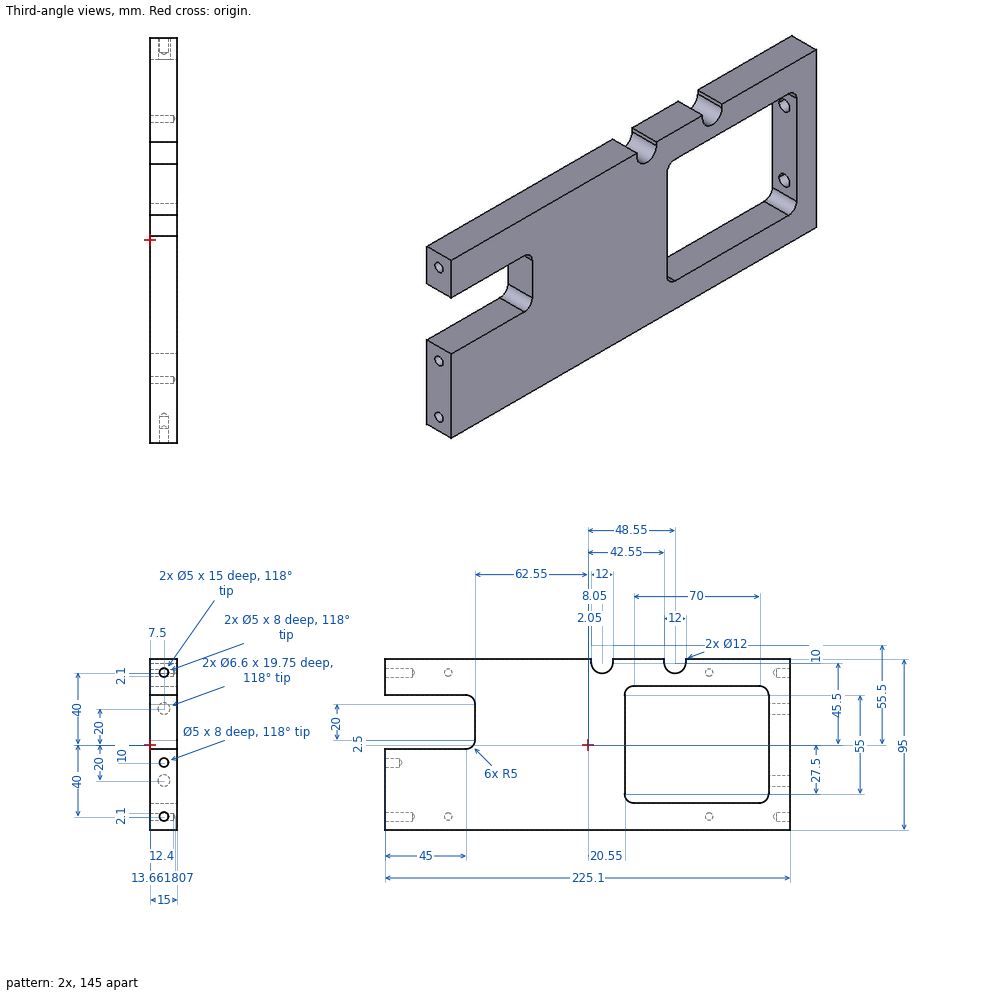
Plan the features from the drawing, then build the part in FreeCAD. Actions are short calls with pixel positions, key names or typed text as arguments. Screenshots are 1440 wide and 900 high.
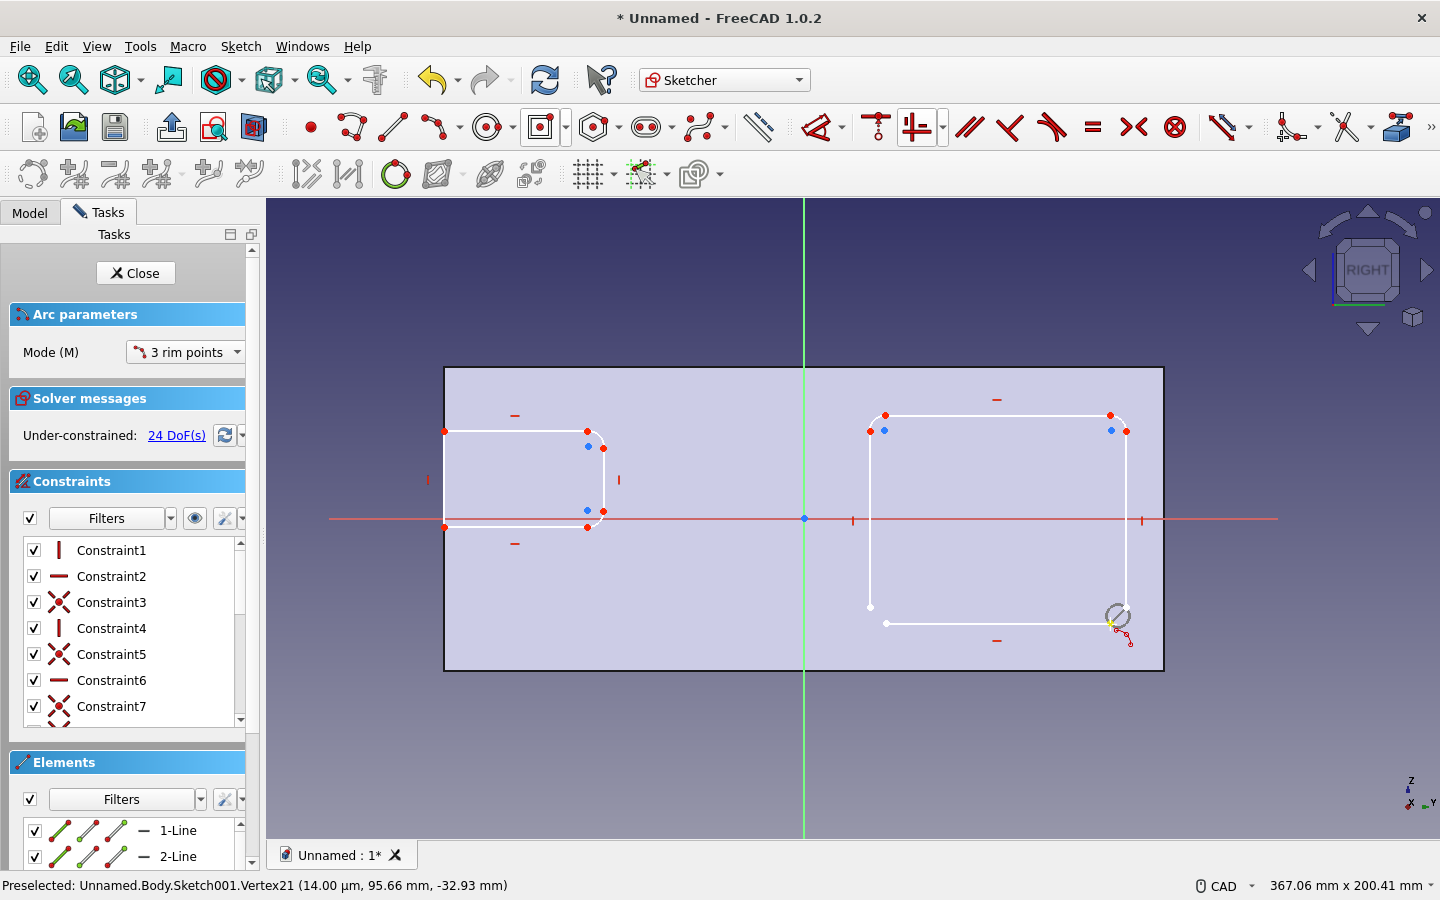
scroll(1121, 618, up, 7)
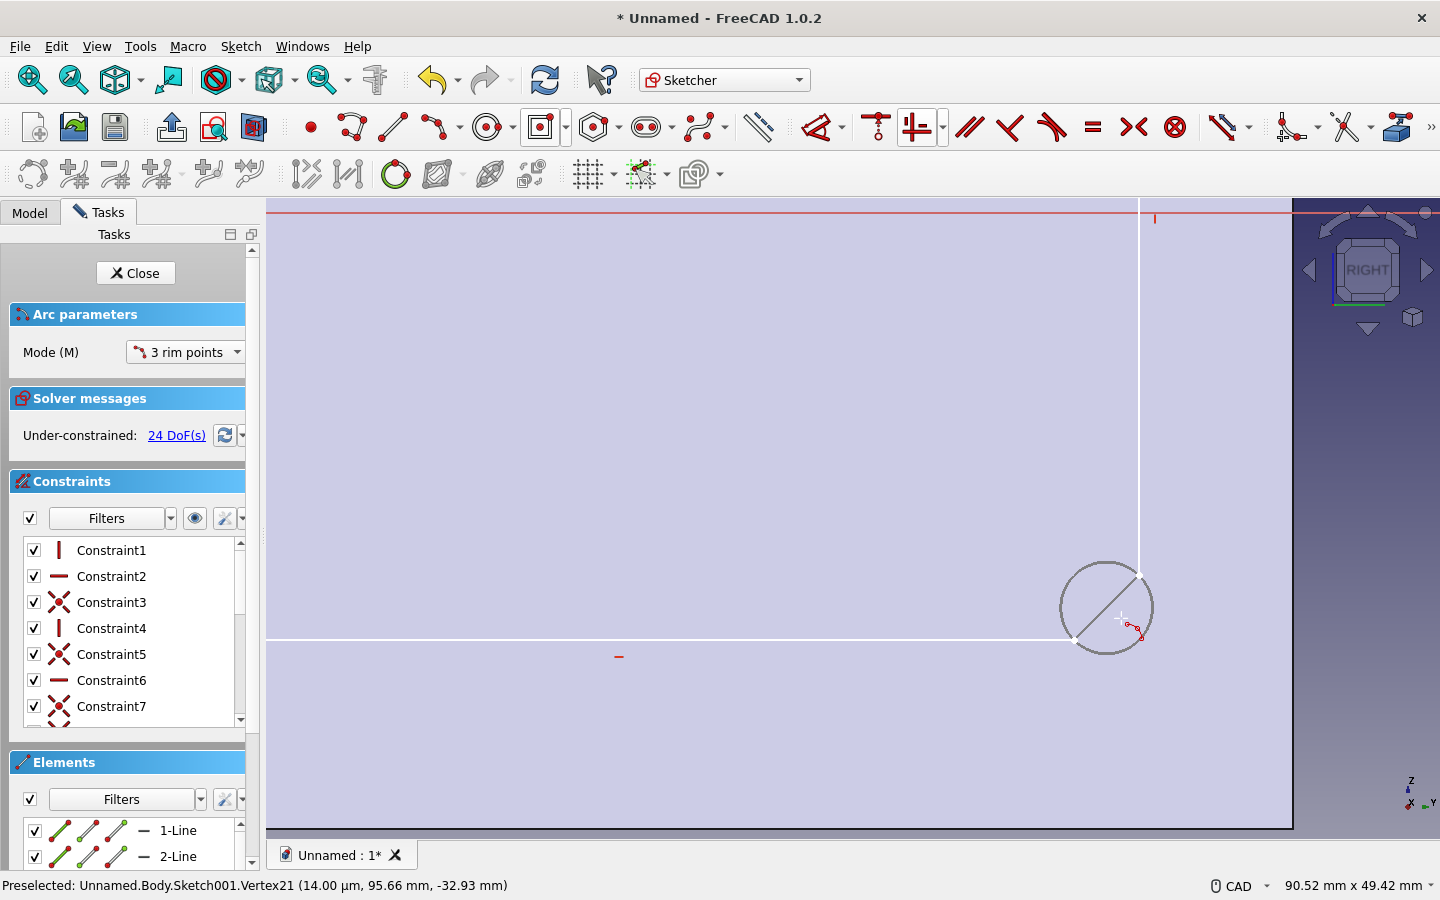
click(1119, 616)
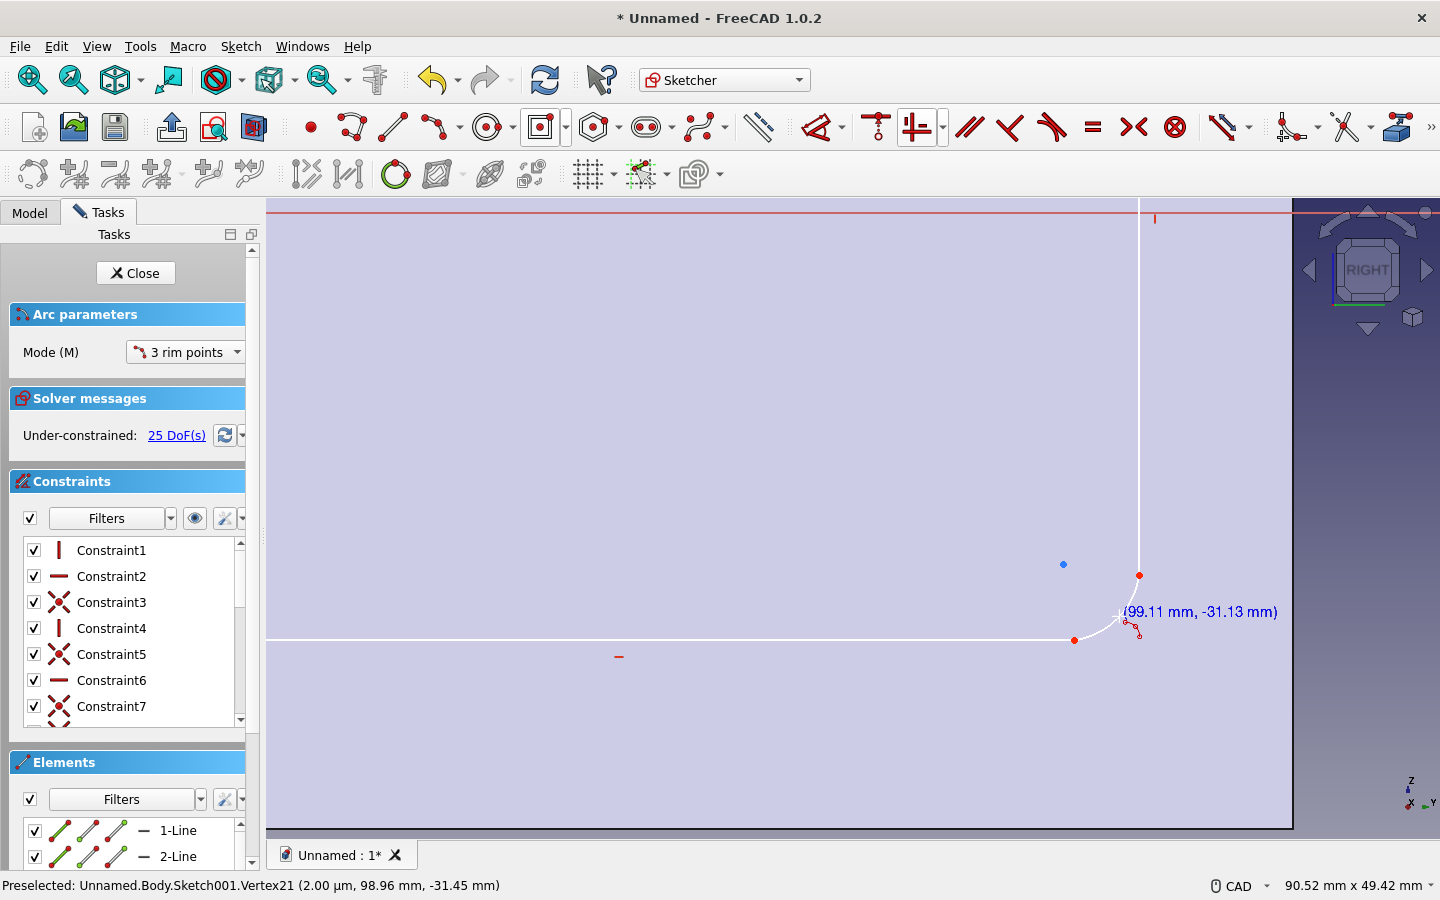
scroll(1121, 618, down, 7)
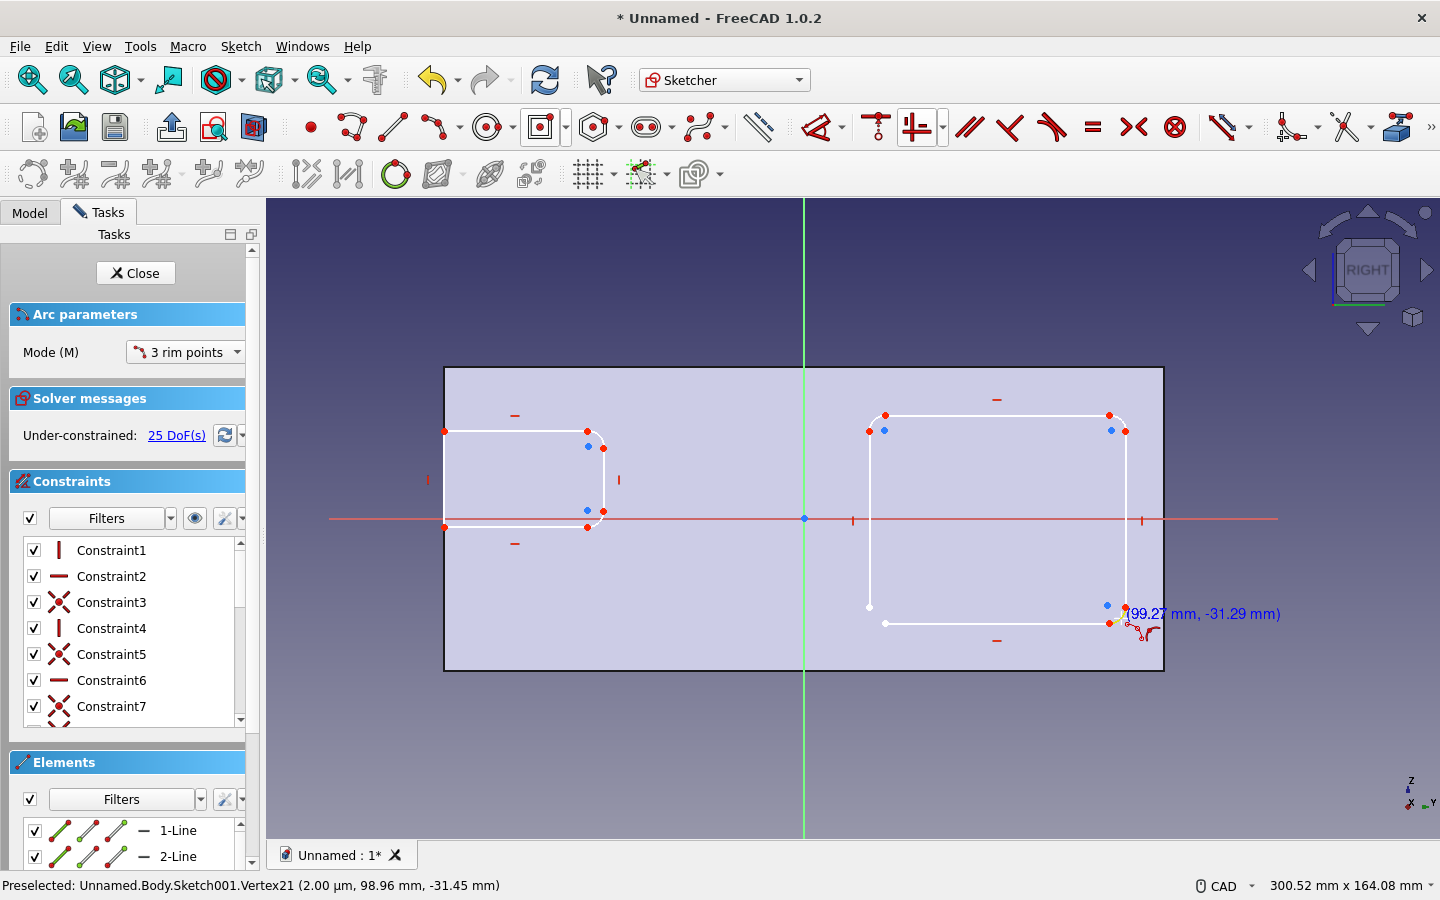
click(886, 624)
click(870, 608)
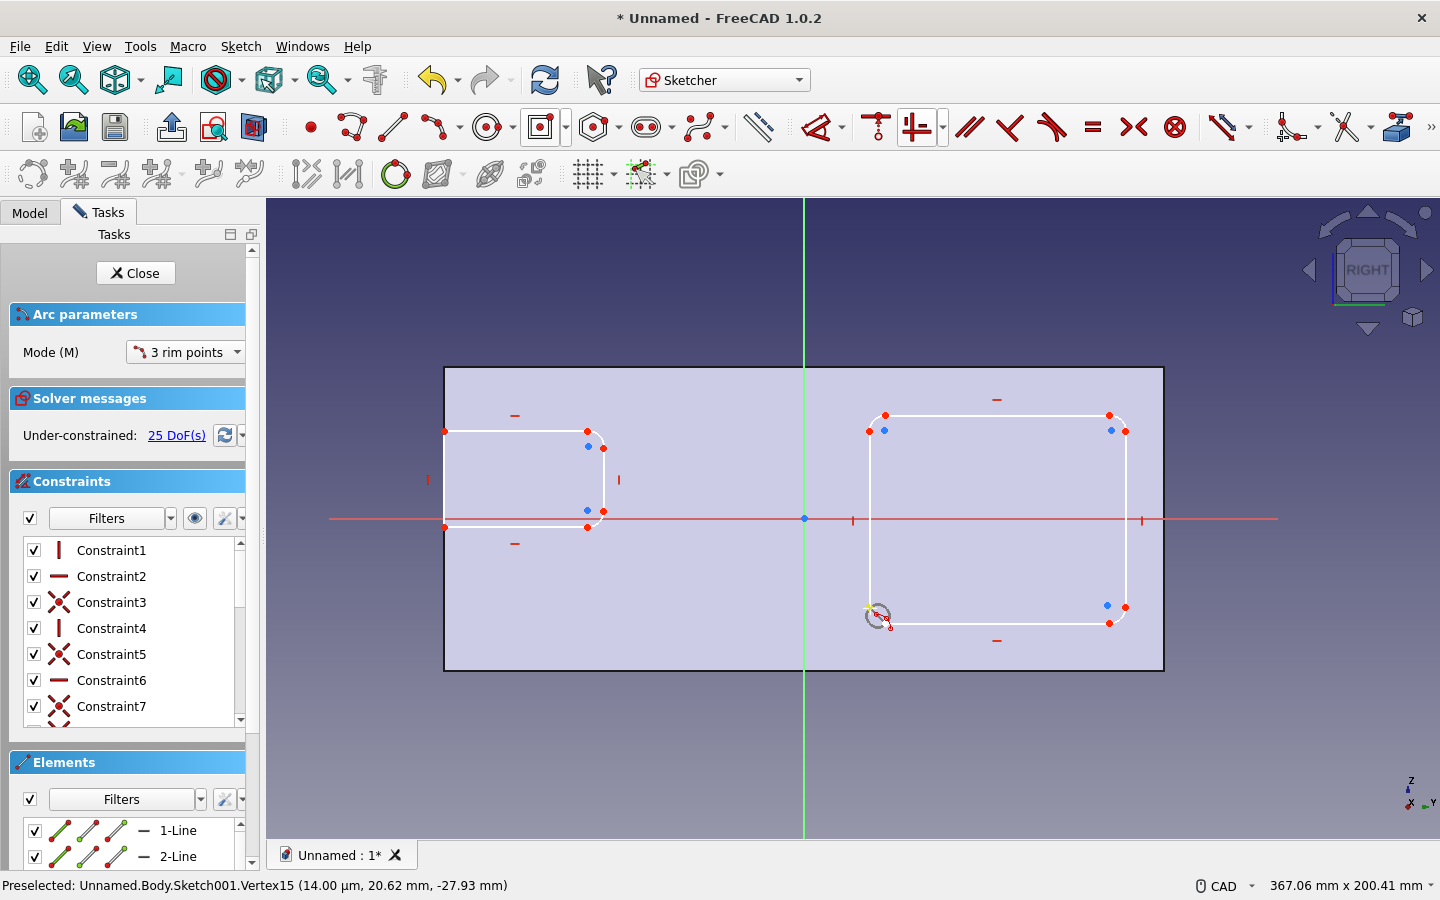
scroll(874, 618, up, 7)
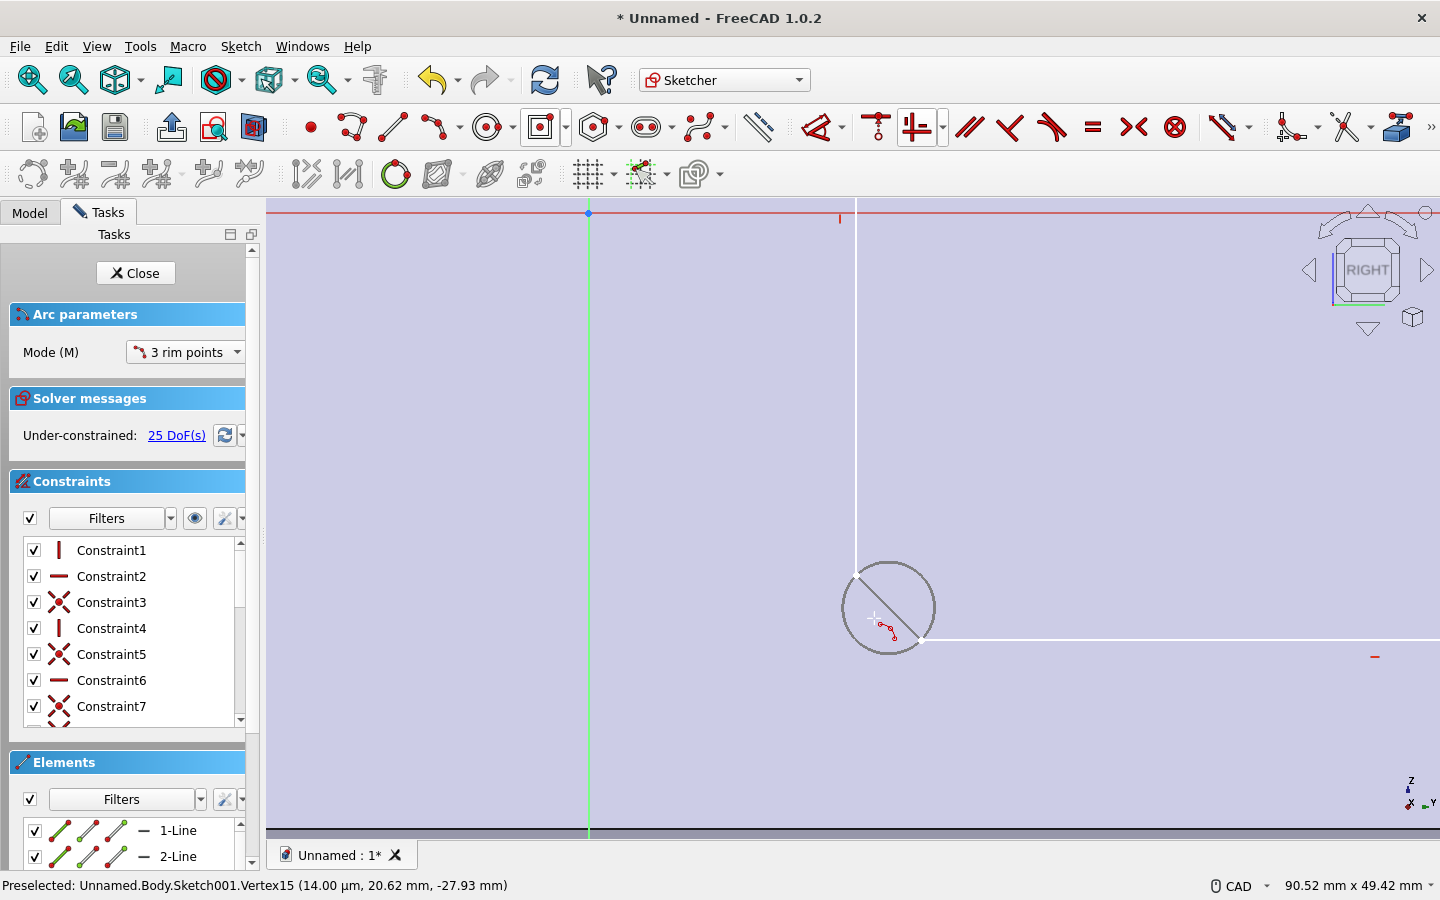
click(874, 616)
key(Escape)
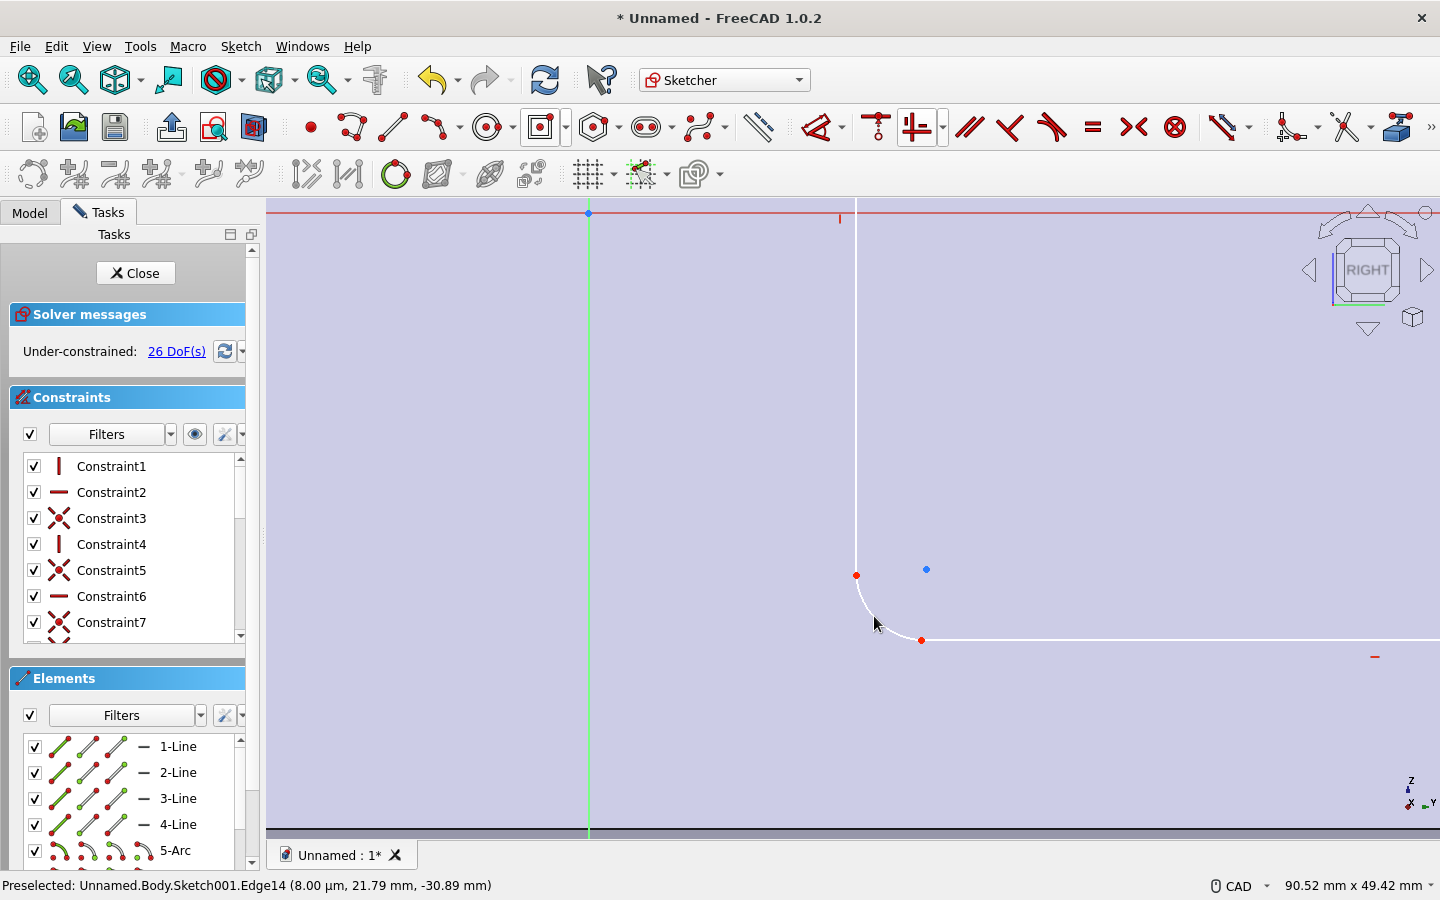
scroll(874, 618, down, 7)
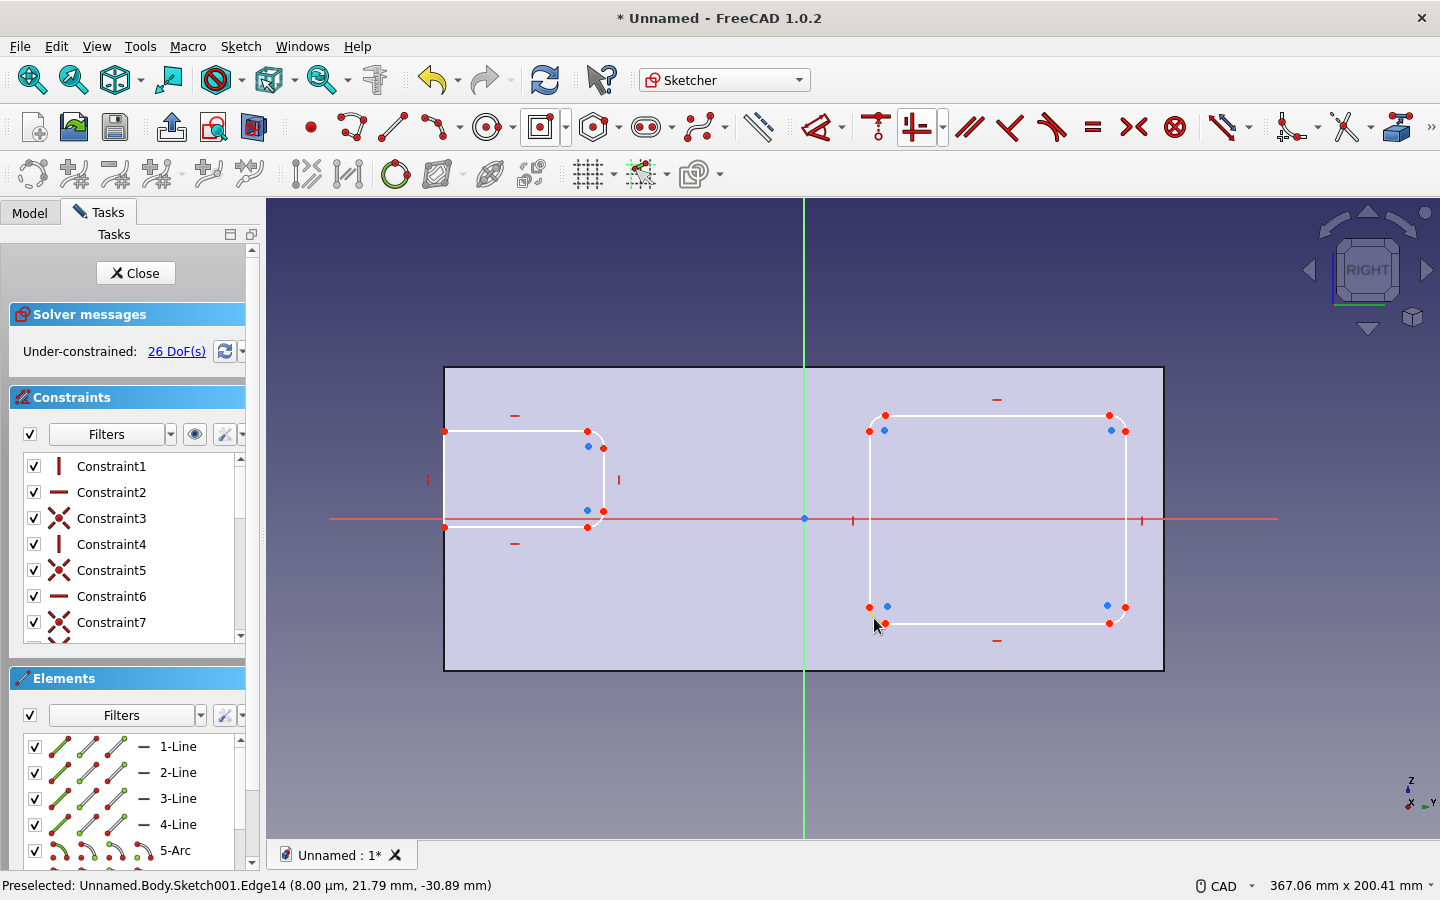
click(604, 467)